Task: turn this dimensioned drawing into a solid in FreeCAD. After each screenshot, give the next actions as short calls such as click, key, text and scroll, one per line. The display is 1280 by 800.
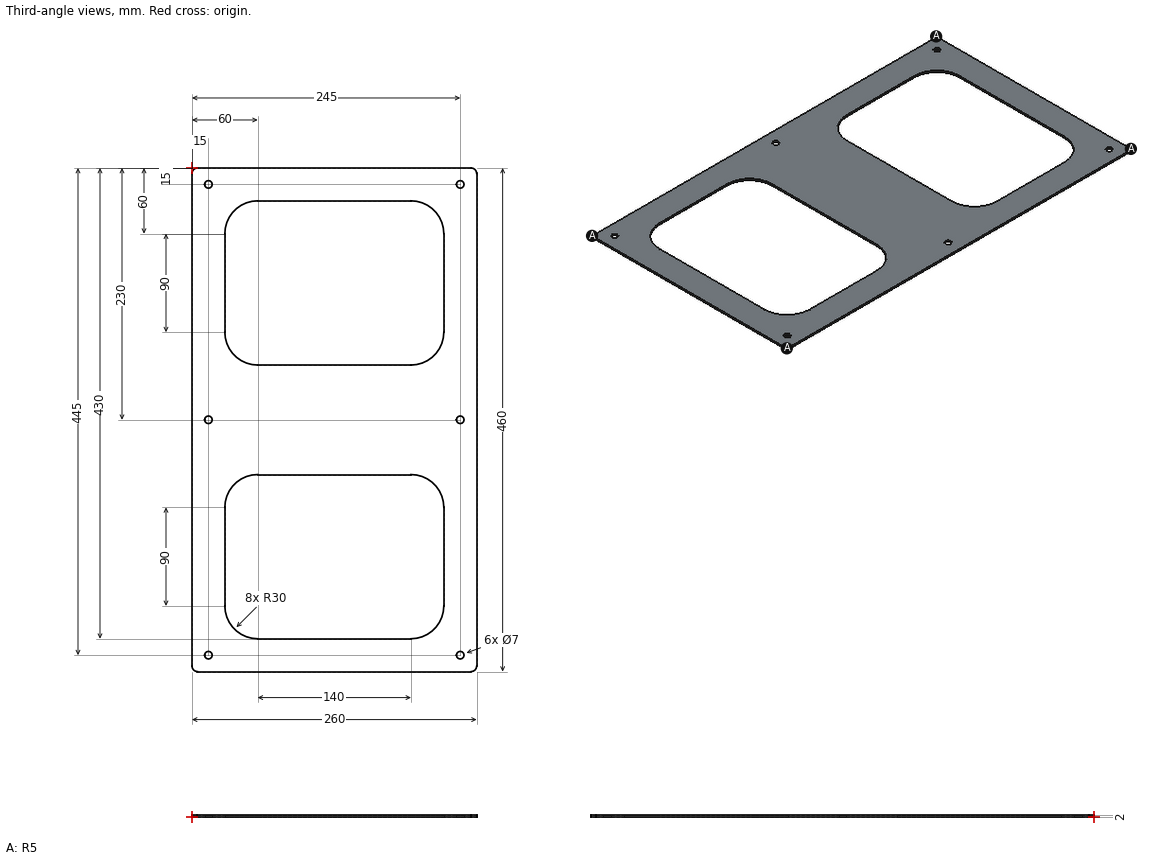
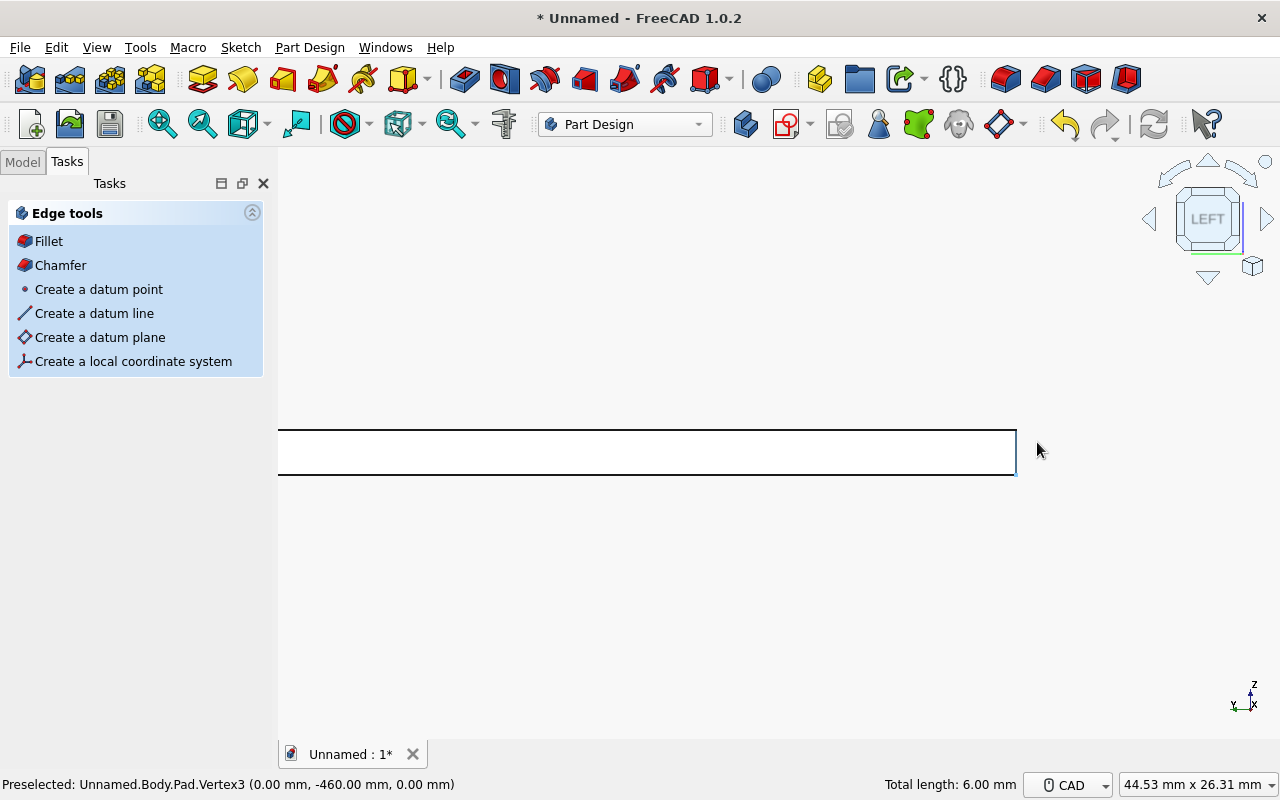
click(164, 124)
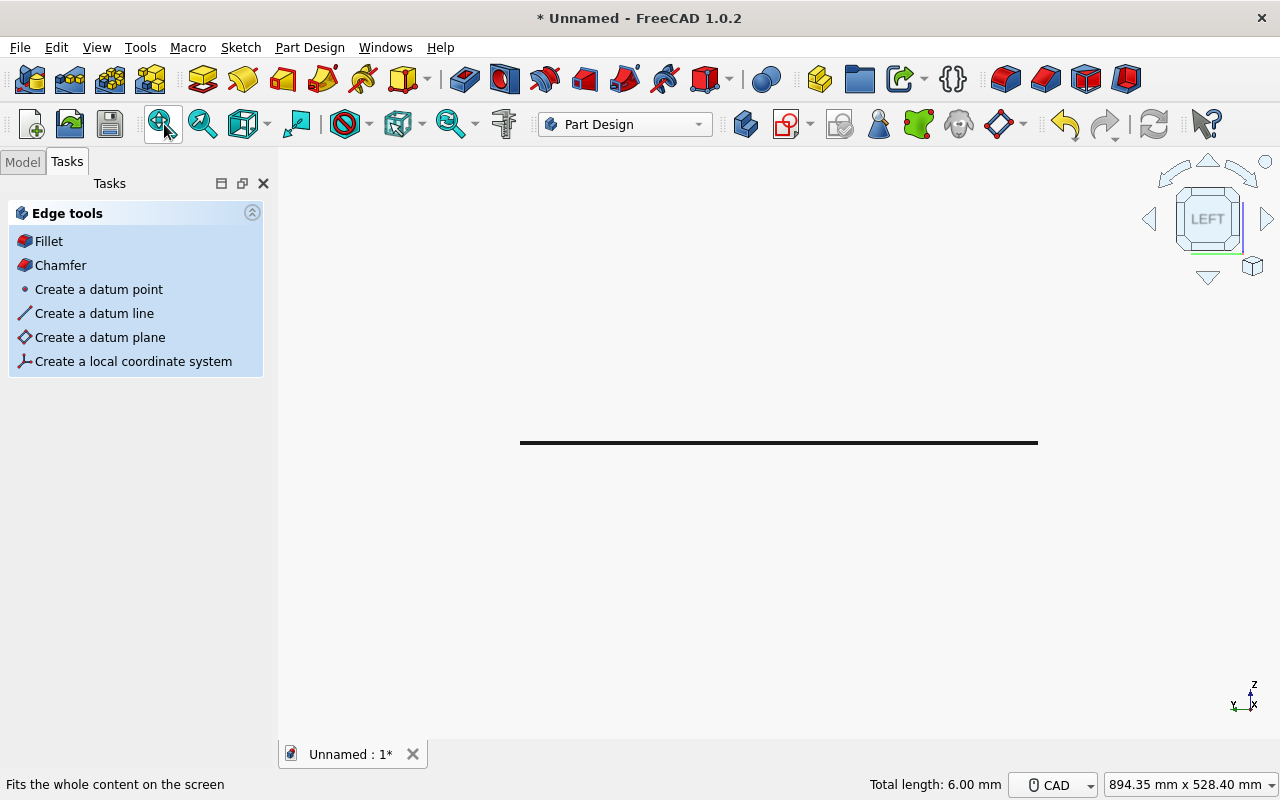
key(v)
key(3)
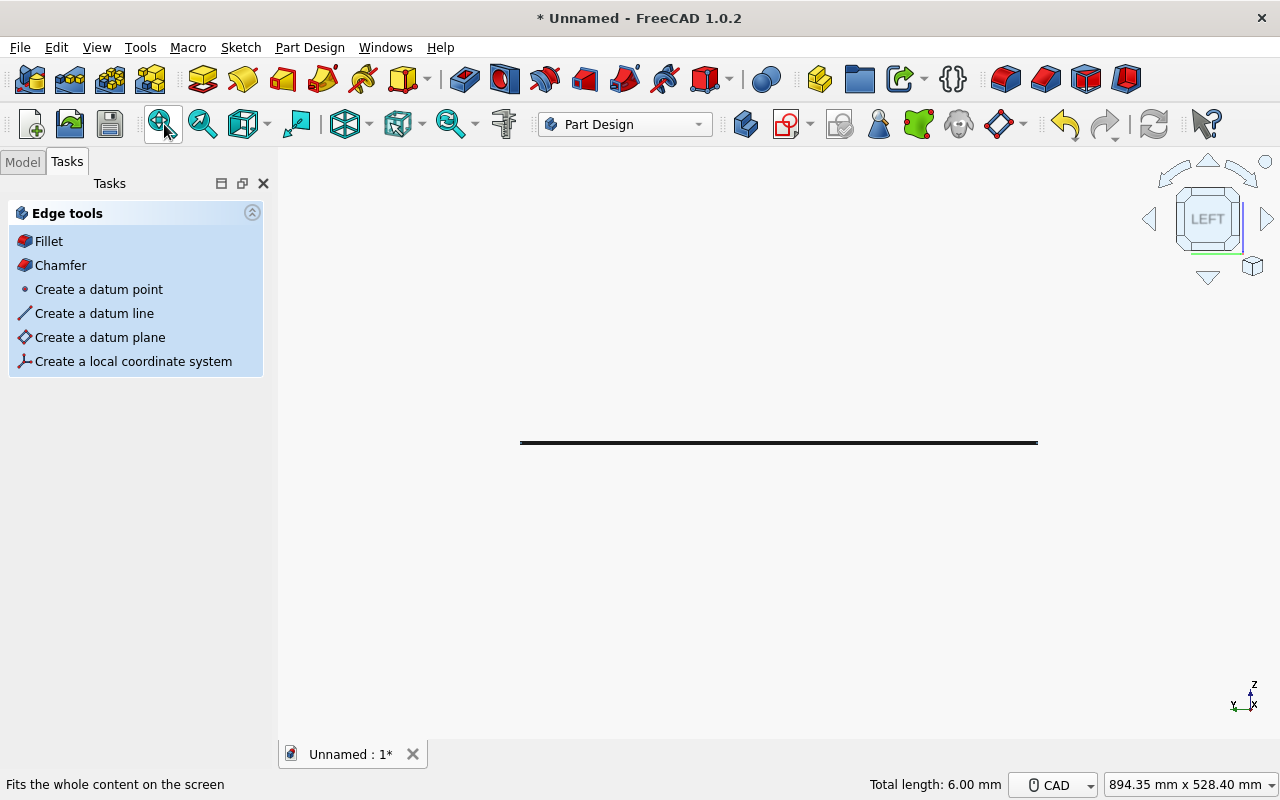
key(0)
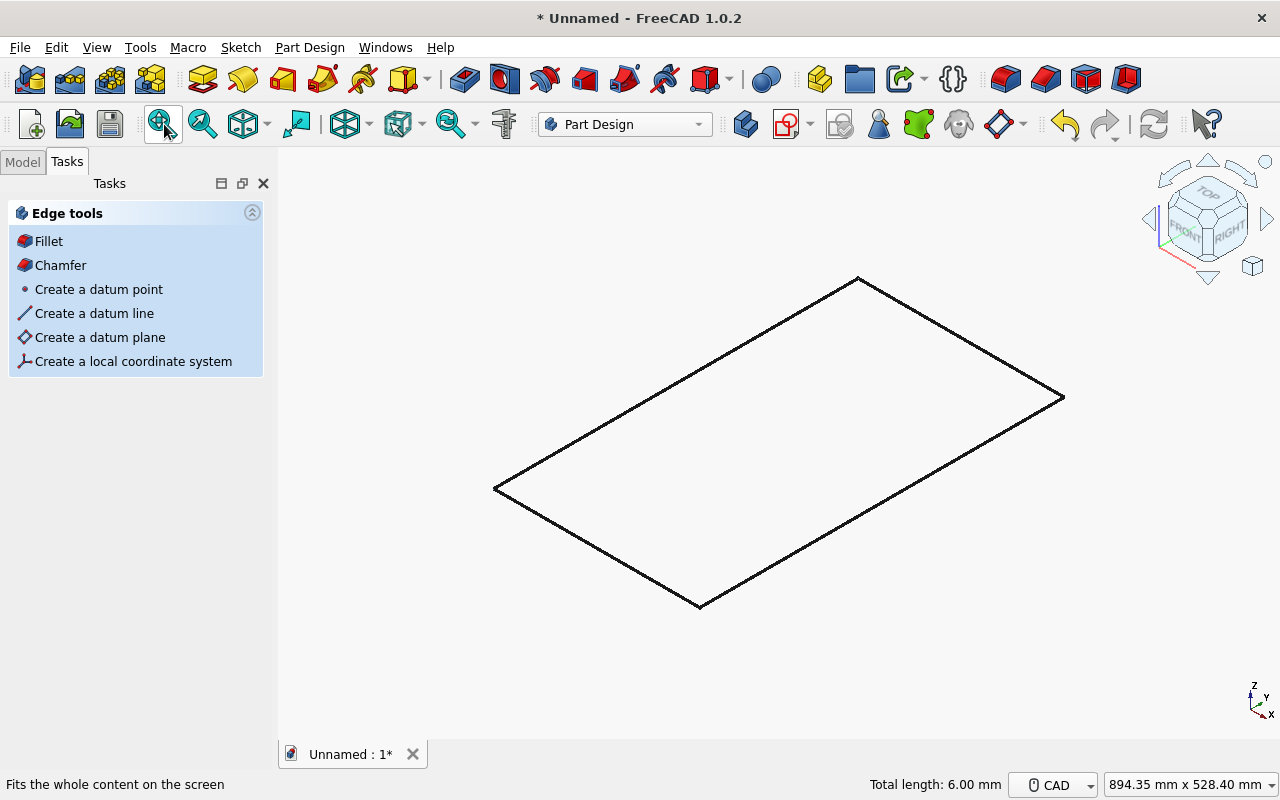
scroll(700, 607, up, 15)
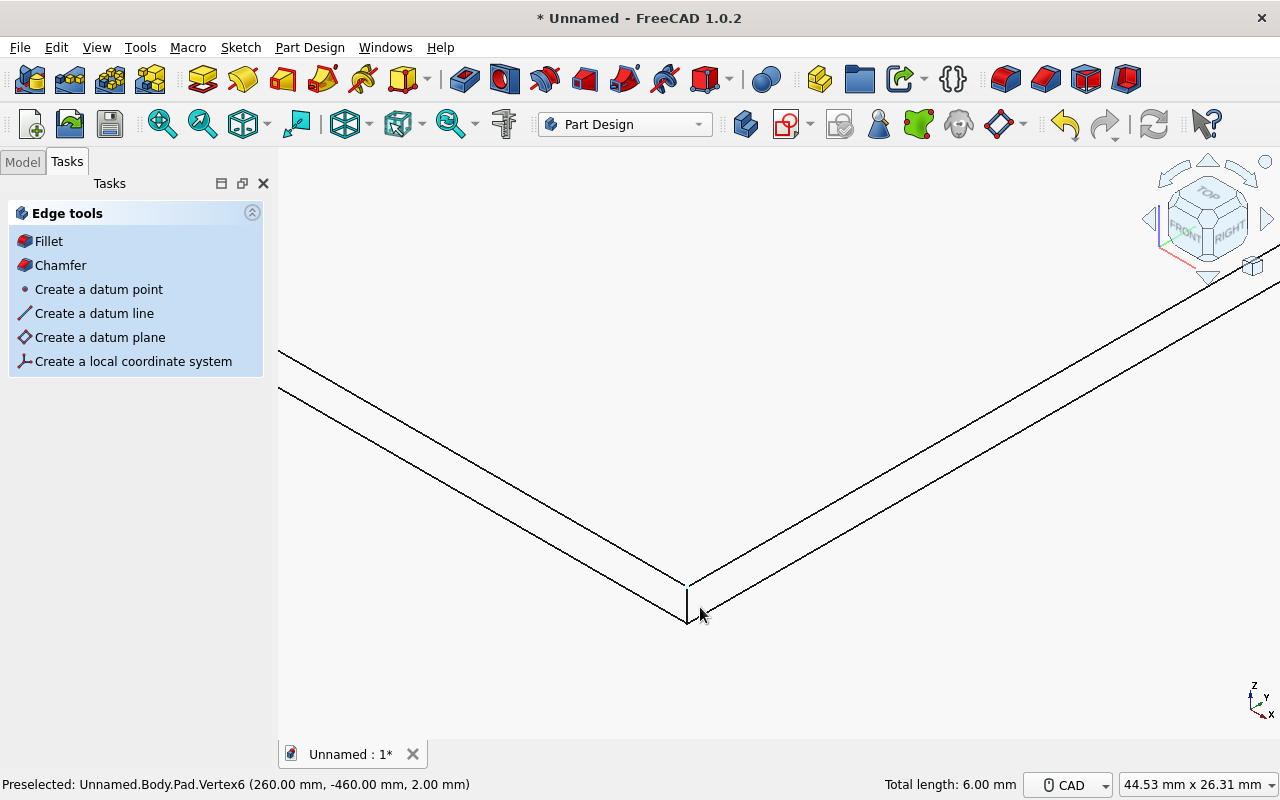
click(687, 604, ctrl)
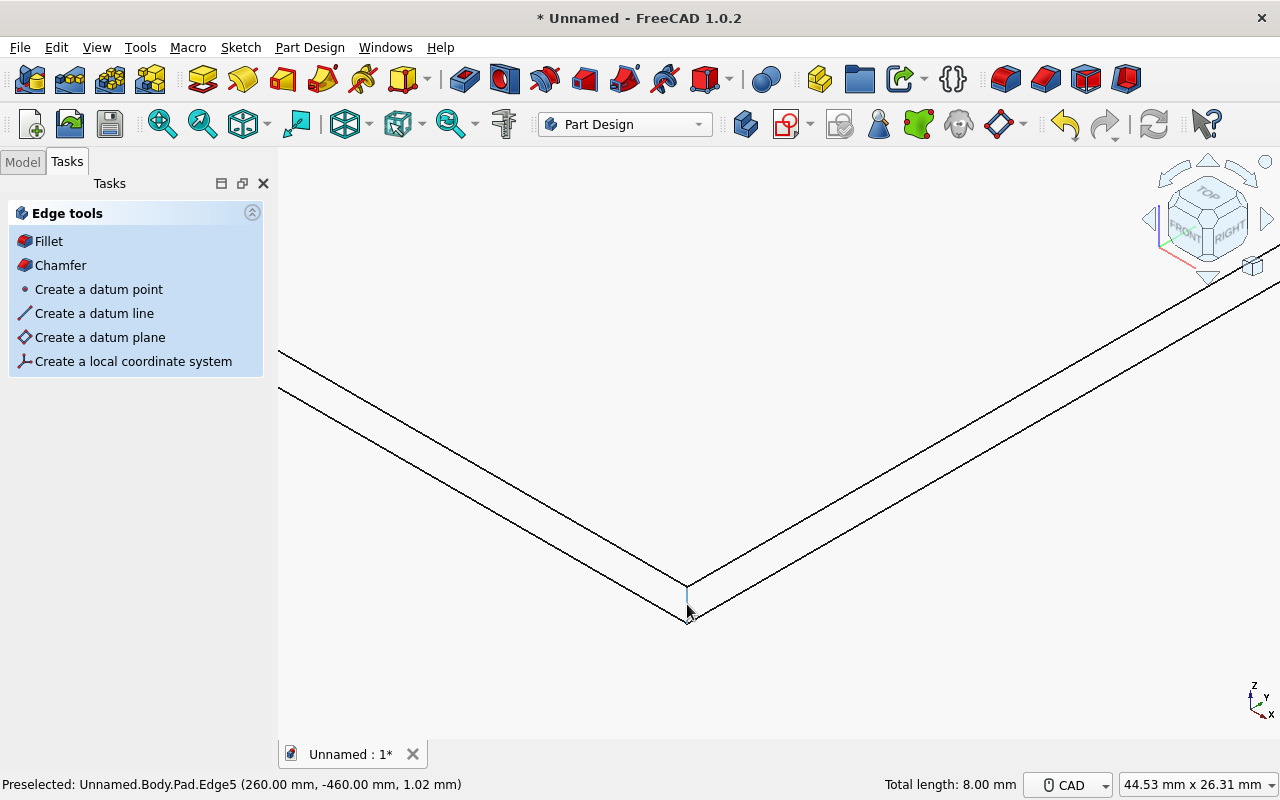
key(v)
key(1)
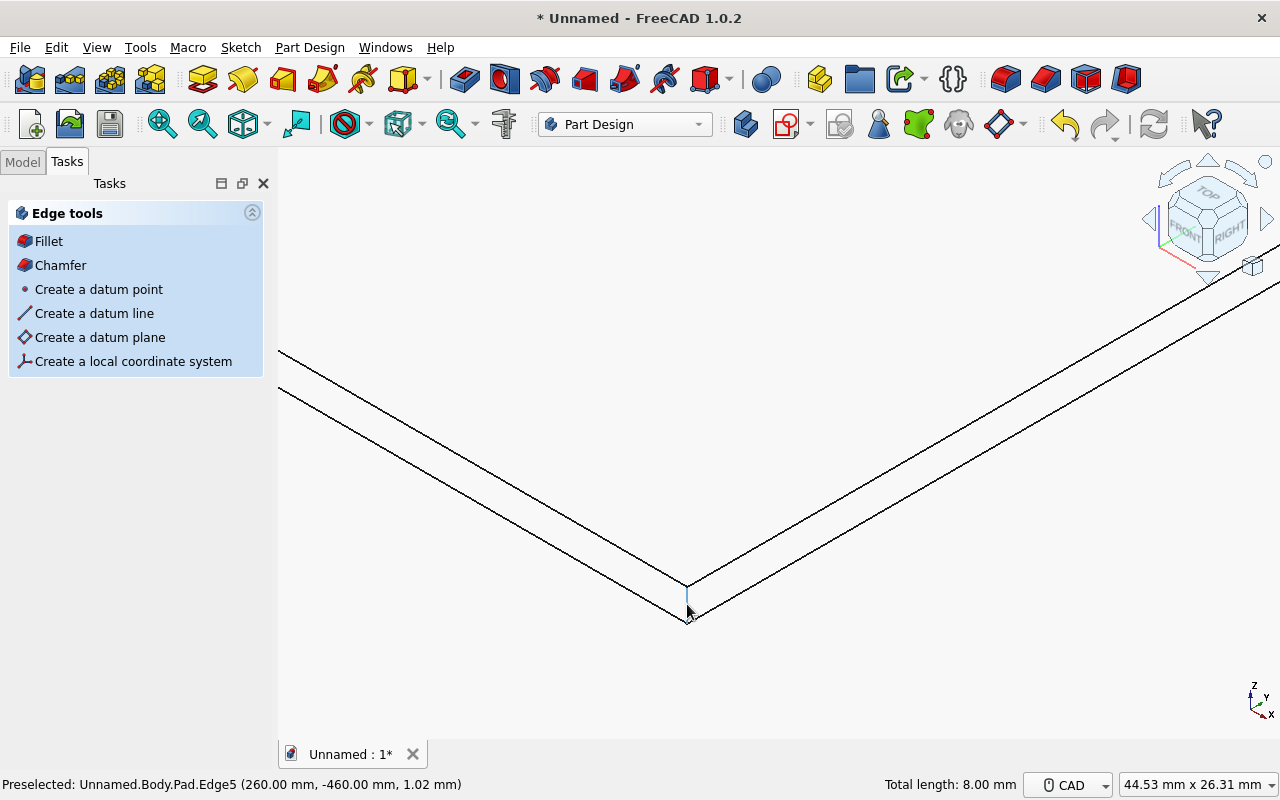
click(1006, 80)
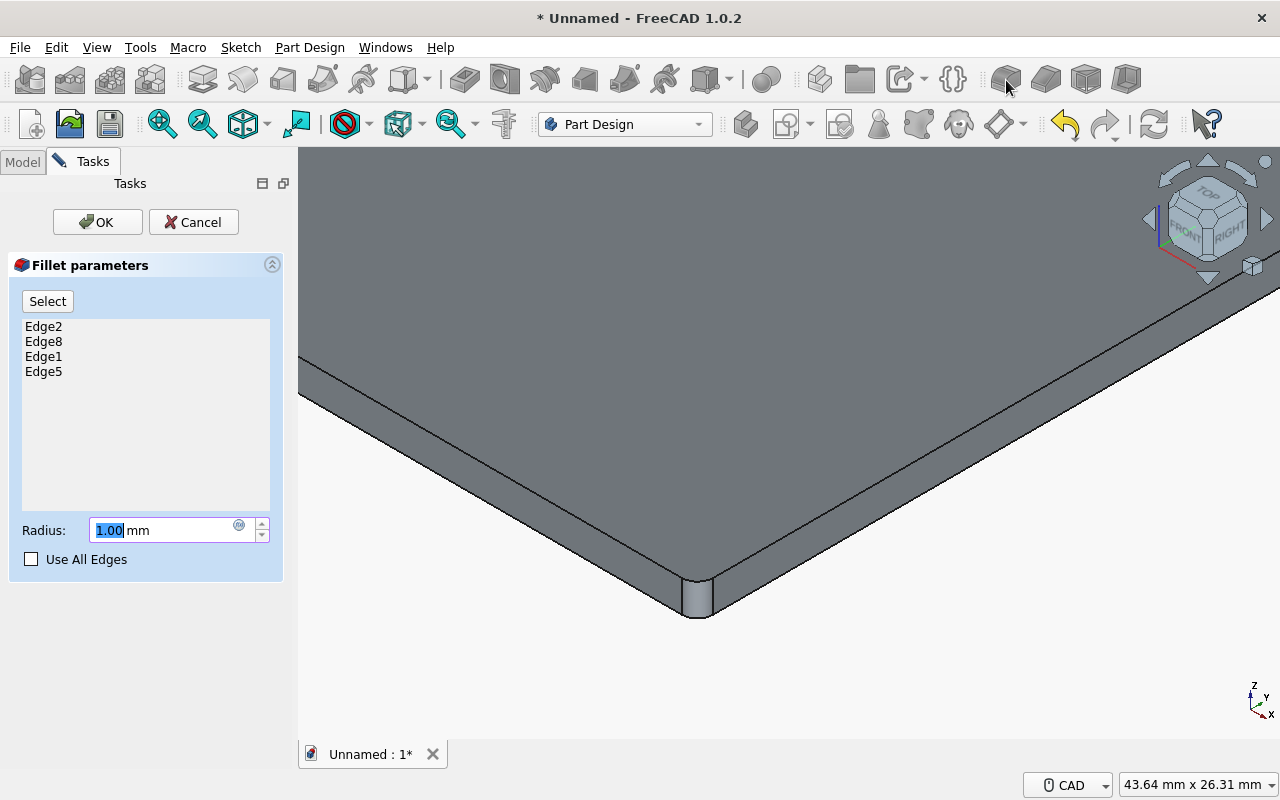
text(5)
key(Tab)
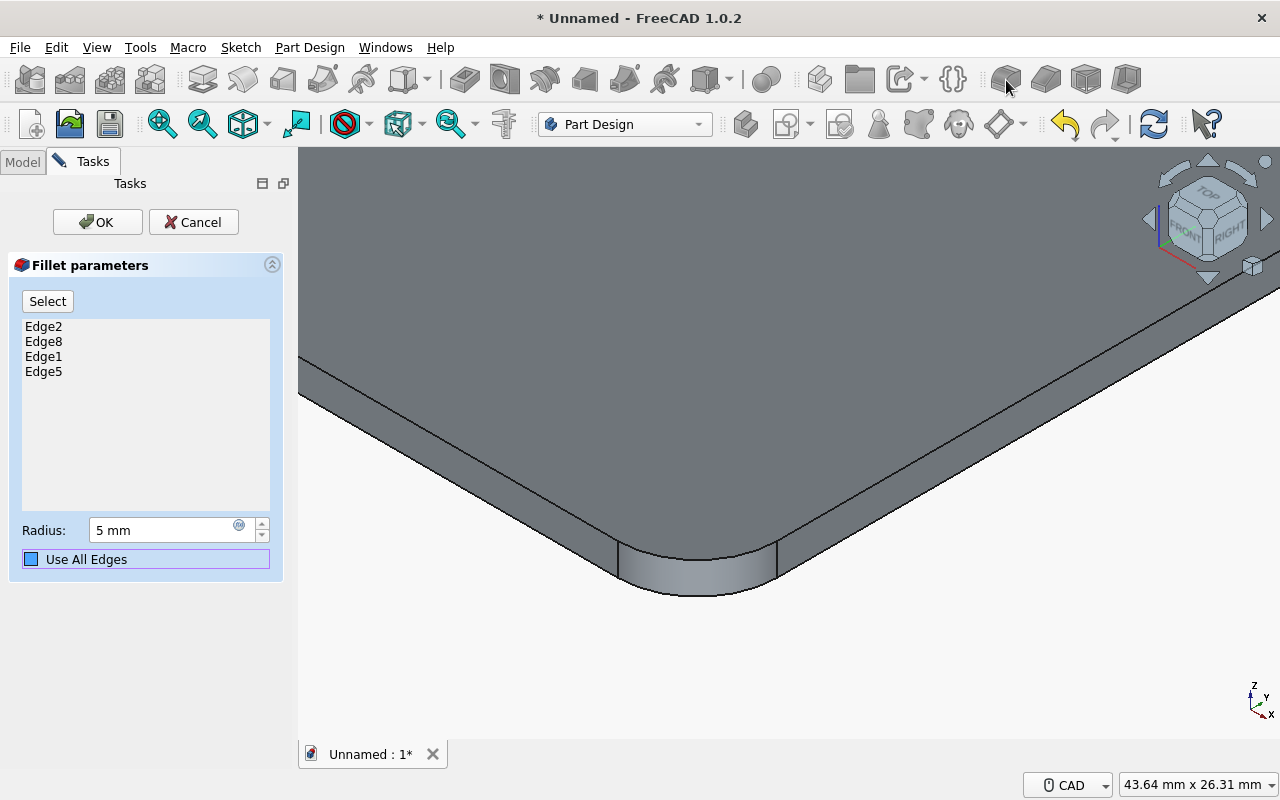
click(98, 222)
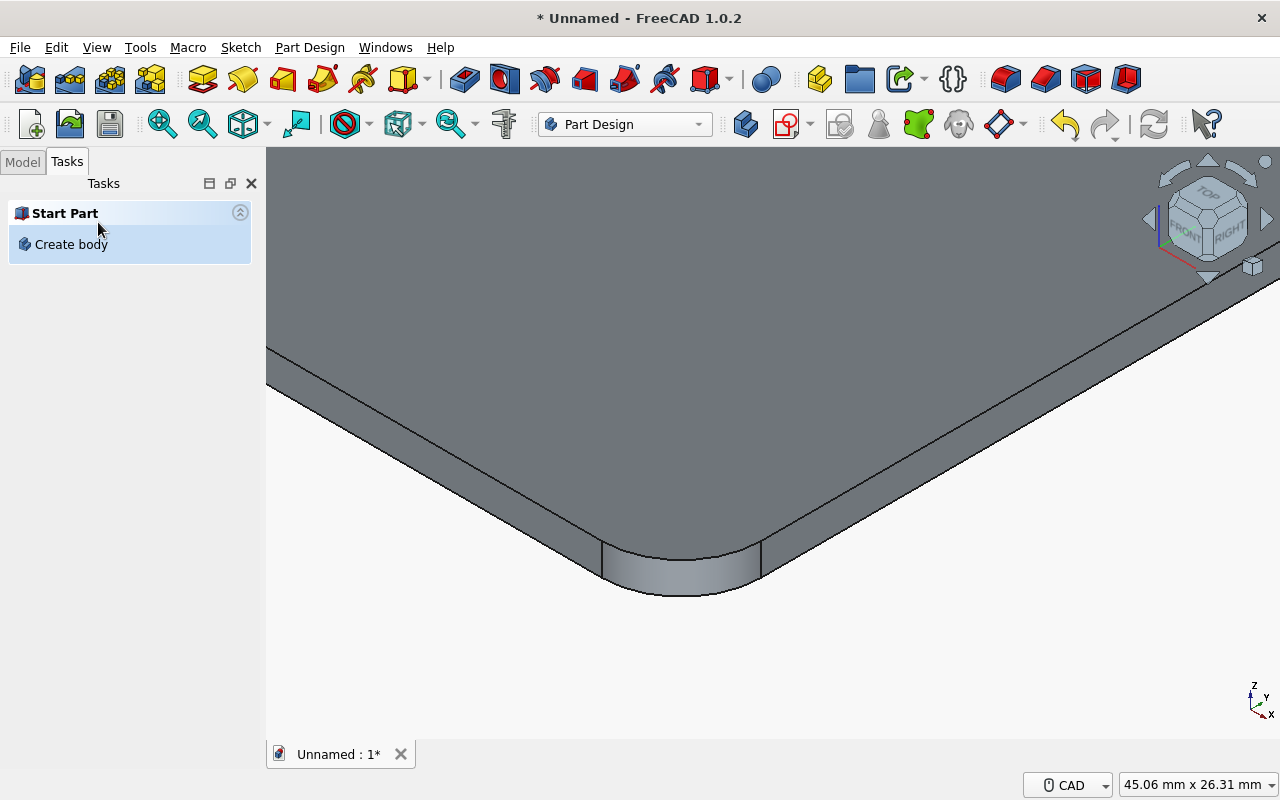
click(164, 124)